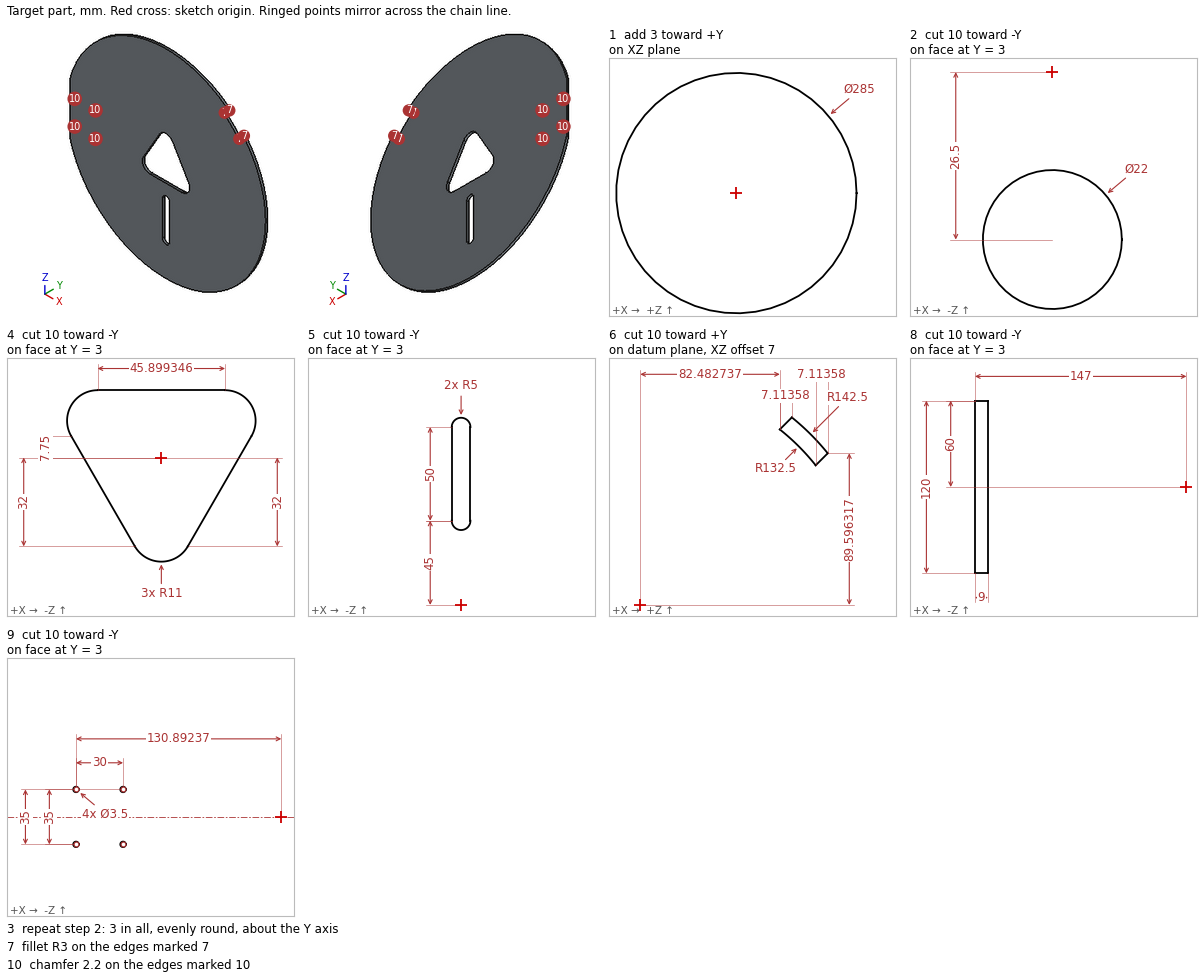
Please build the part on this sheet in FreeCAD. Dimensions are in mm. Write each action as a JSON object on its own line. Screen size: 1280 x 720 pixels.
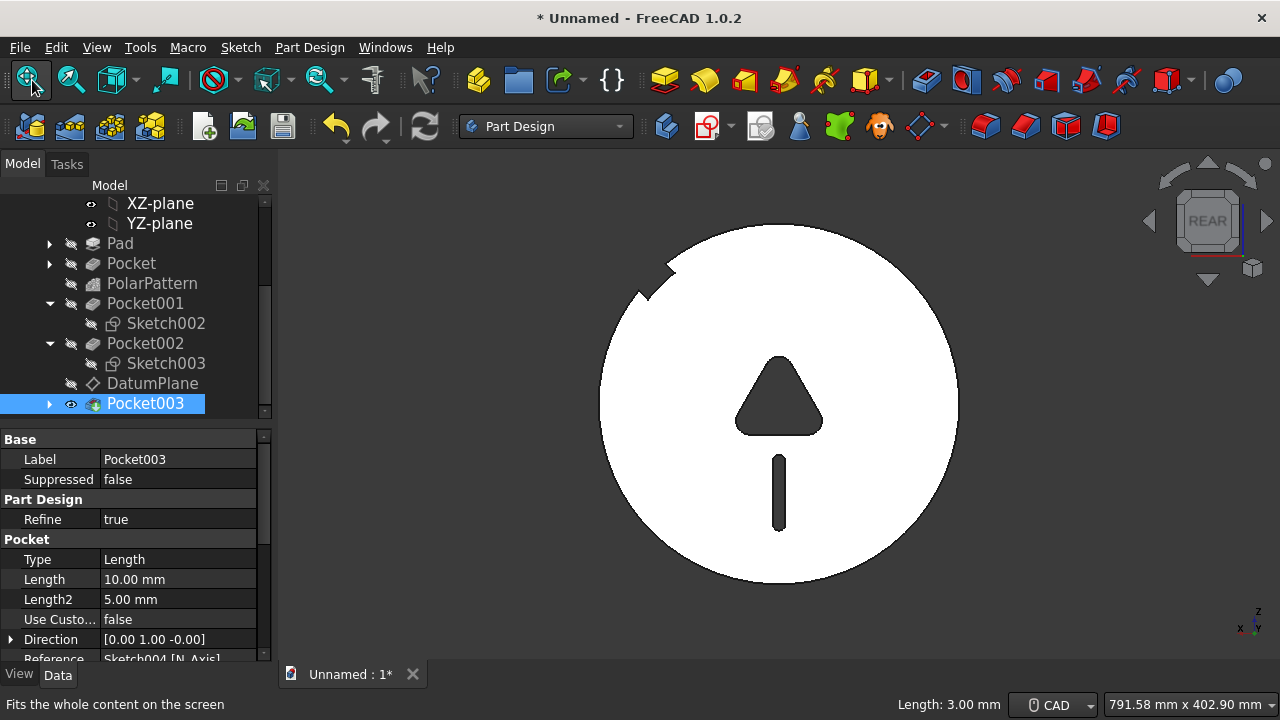
{"action": "scroll", "coordinate": [675, 272], "scroll_direction": "up", "scroll_amount": 12}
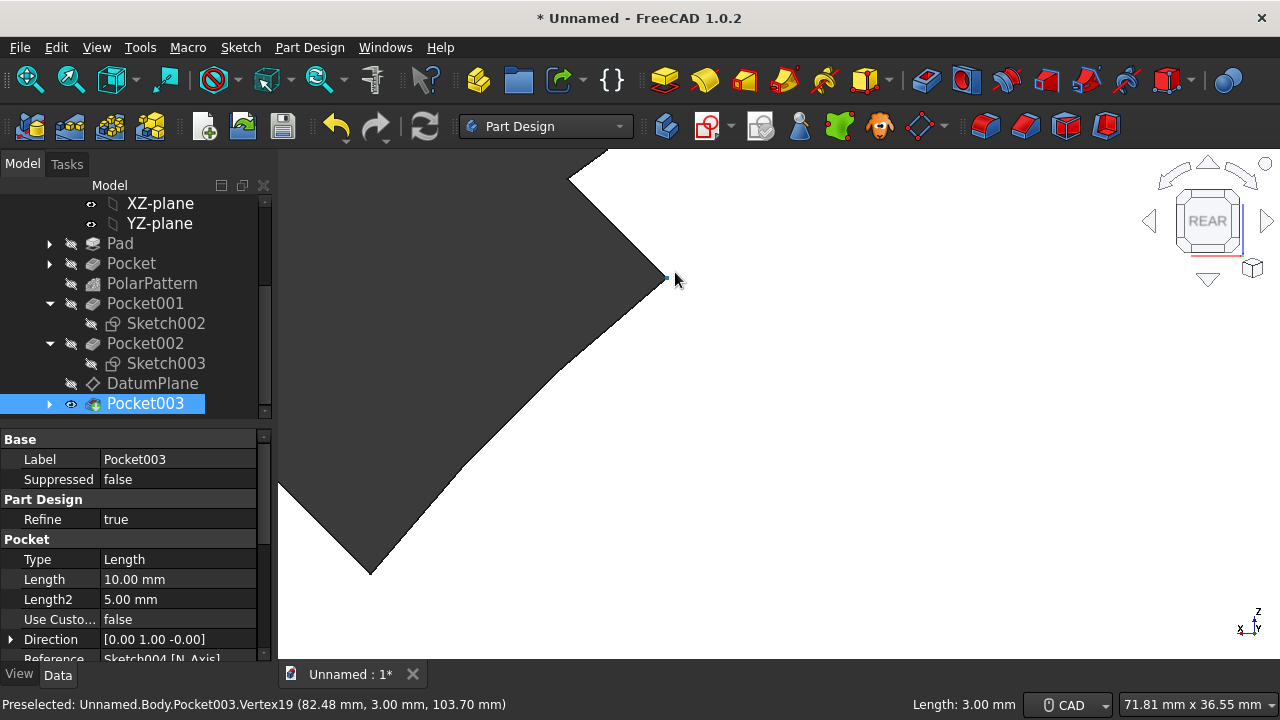
{"action": "left_click", "coordinate": [32, 80]}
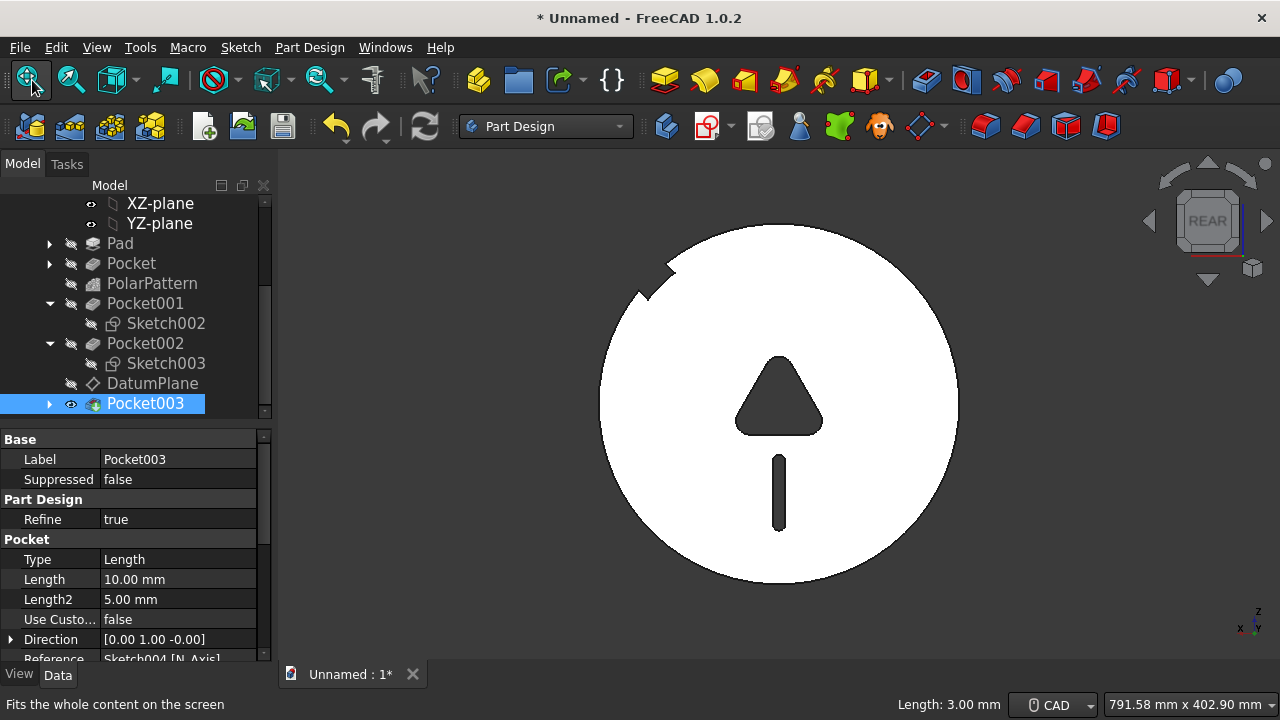
{"action": "key", "text": "6"}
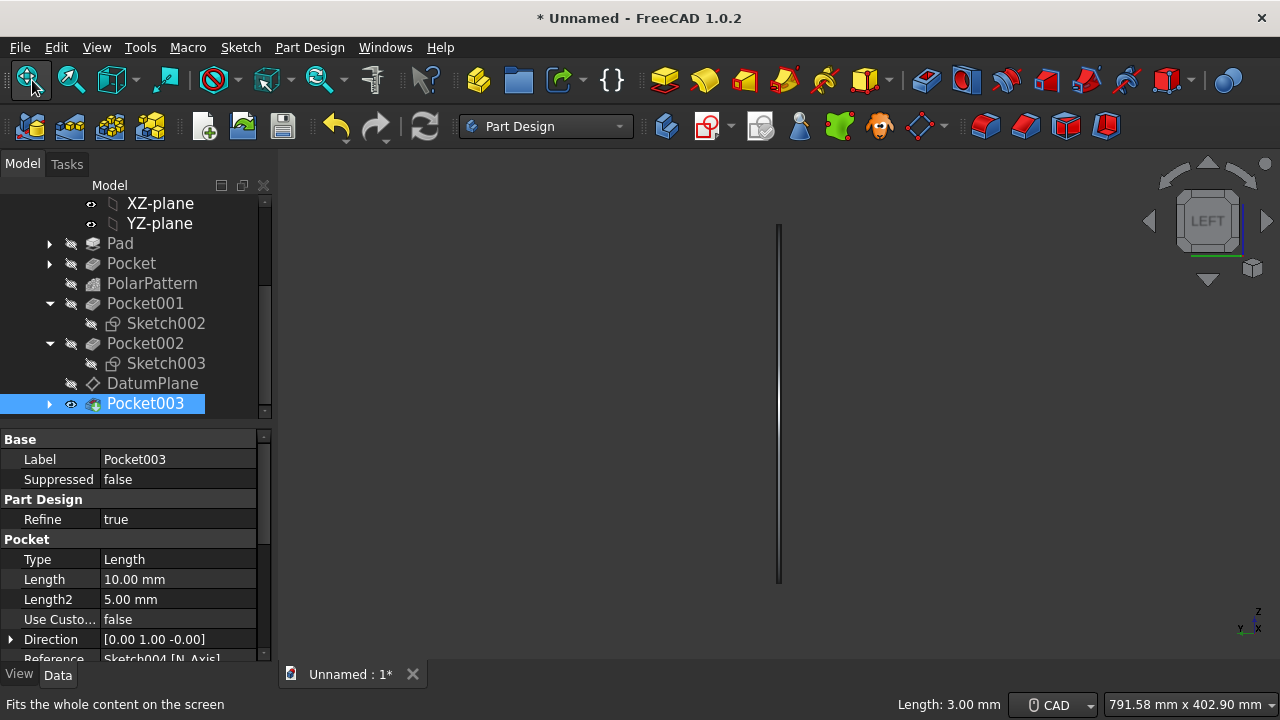
{"action": "scroll", "coordinate": [779, 272], "scroll_direction": "up", "scroll_amount": 12}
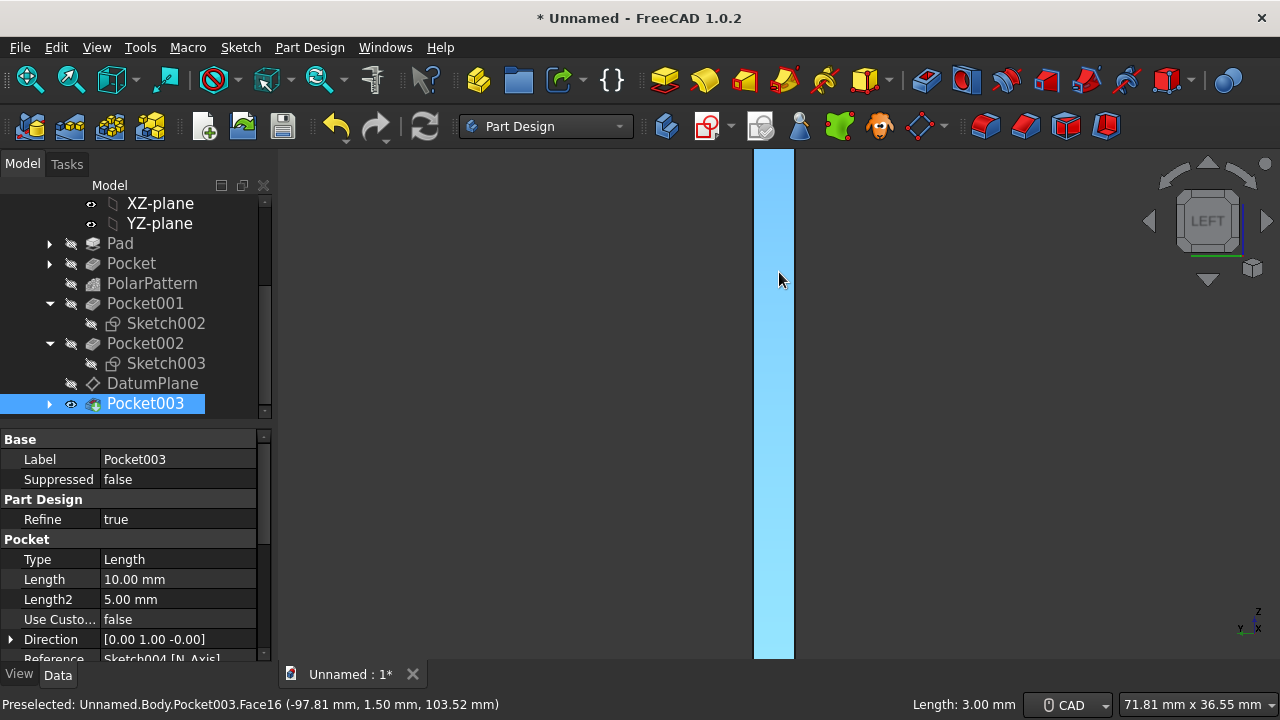
{"action": "left_click", "coordinate": [32, 80]}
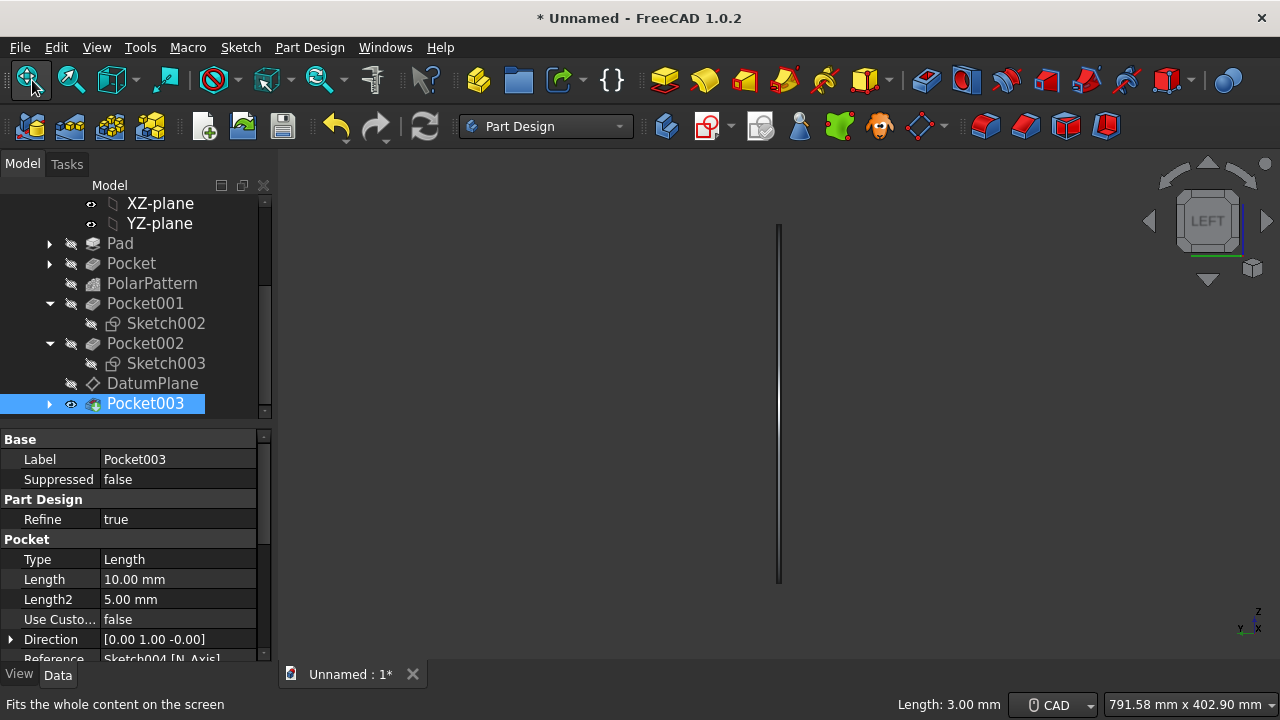
{"action": "key", "text": "v 3"}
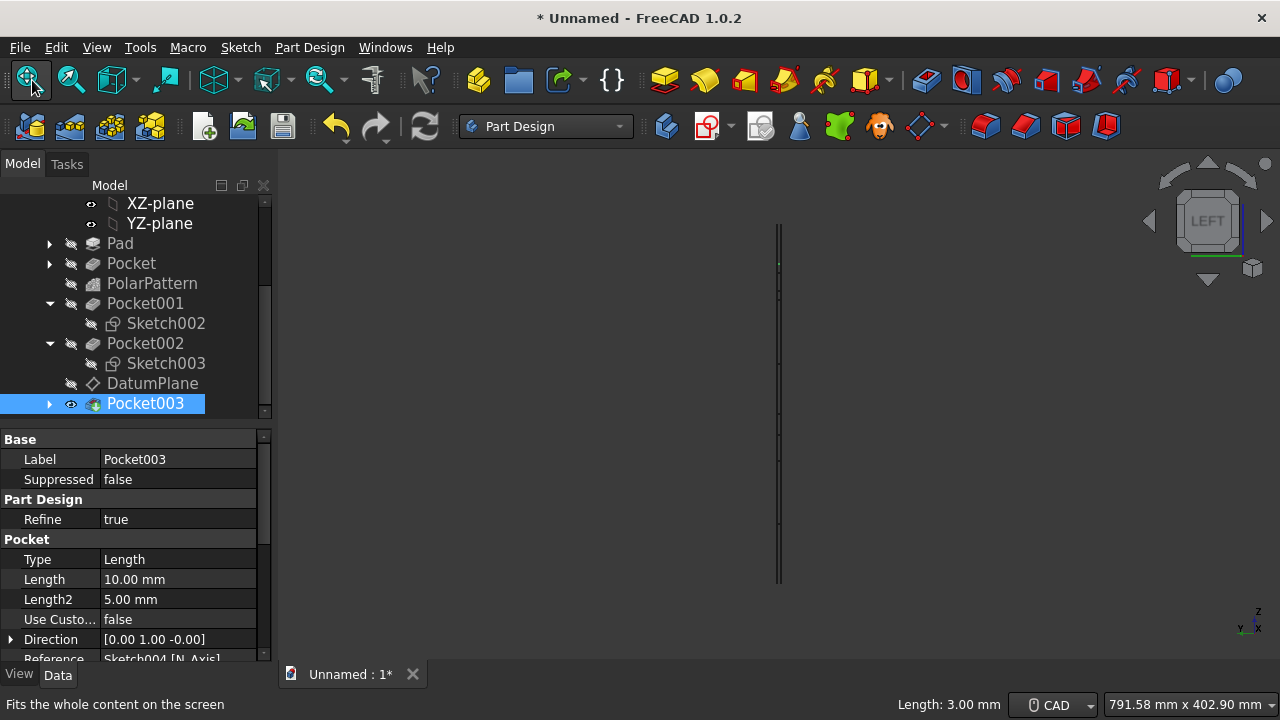
{"action": "key", "text": "0"}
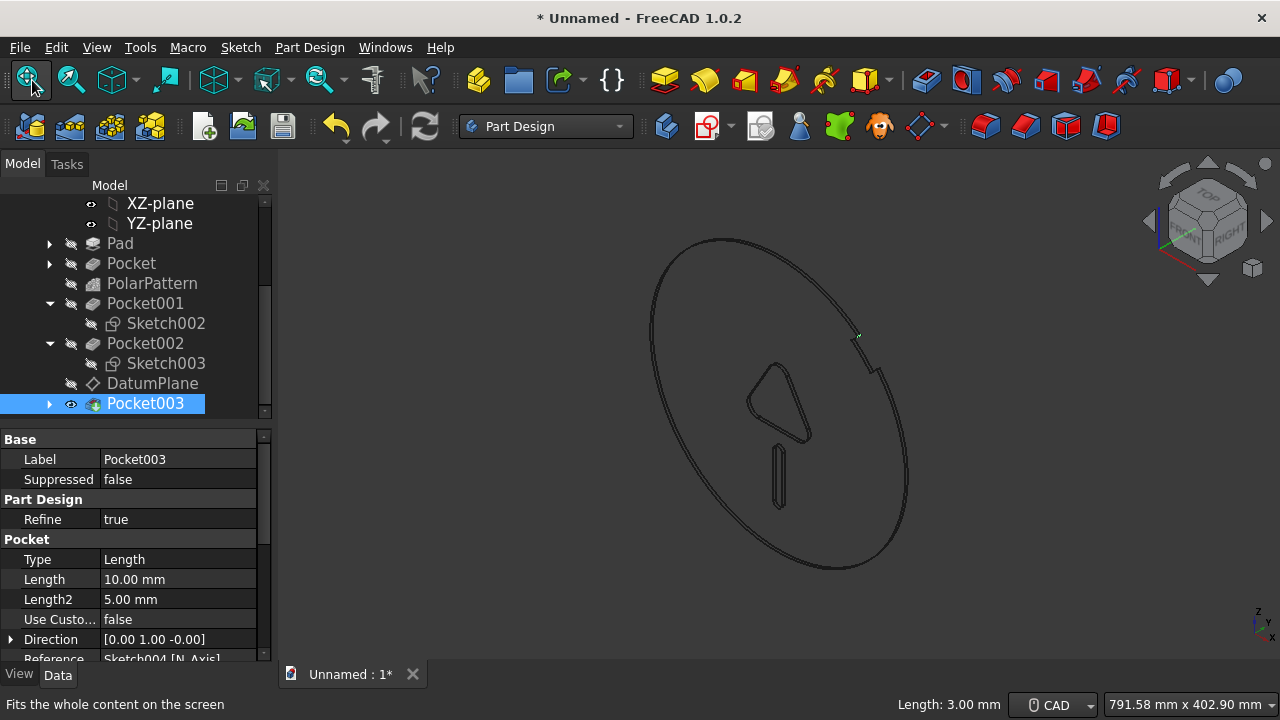
{"action": "scroll", "coordinate": [853, 338], "scroll_direction": "up", "scroll_amount": 12}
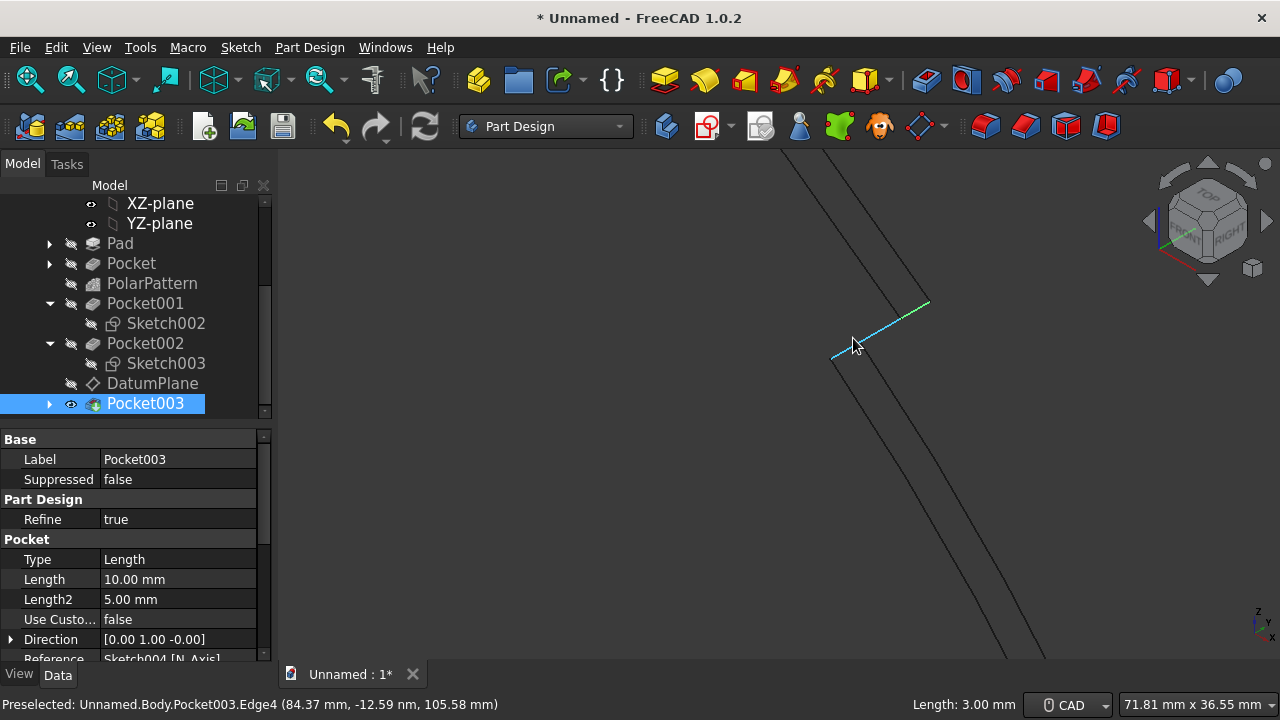
{"action": "key", "text": "v f"}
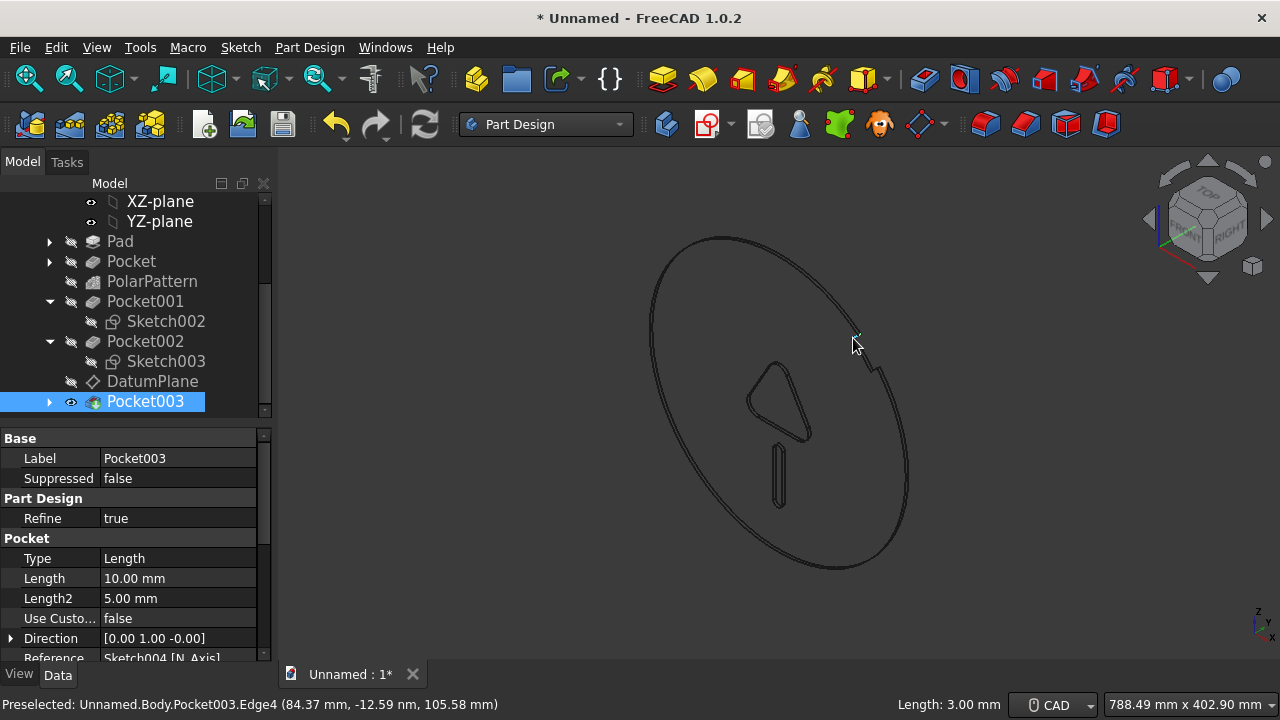
{"action": "key", "text": "2"}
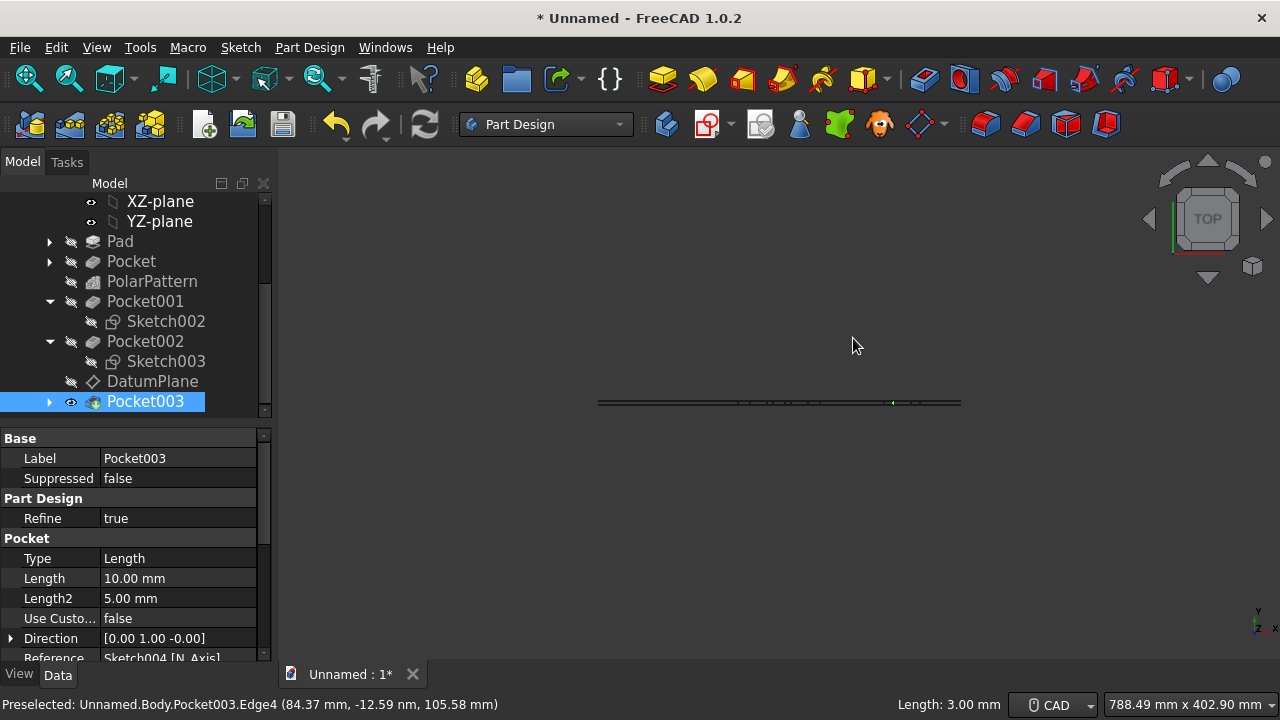
{"action": "left_click", "coordinate": [30, 80]}